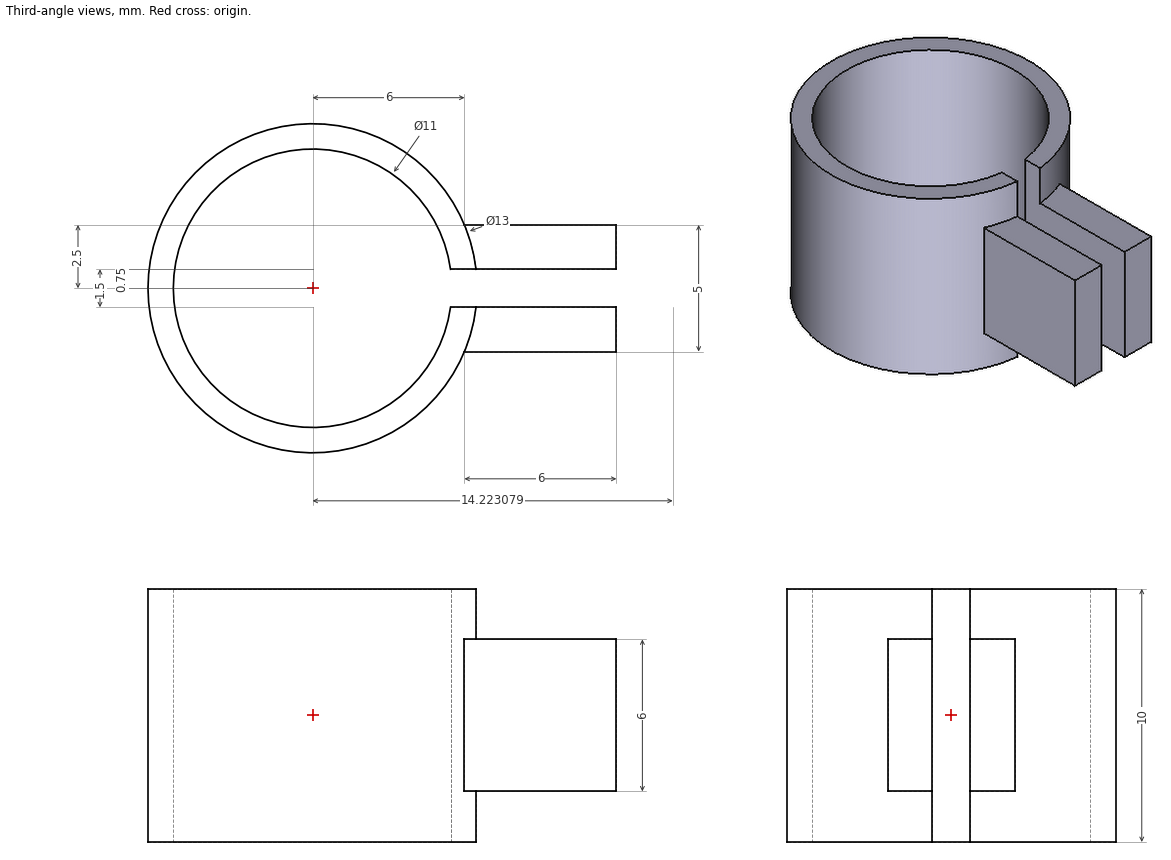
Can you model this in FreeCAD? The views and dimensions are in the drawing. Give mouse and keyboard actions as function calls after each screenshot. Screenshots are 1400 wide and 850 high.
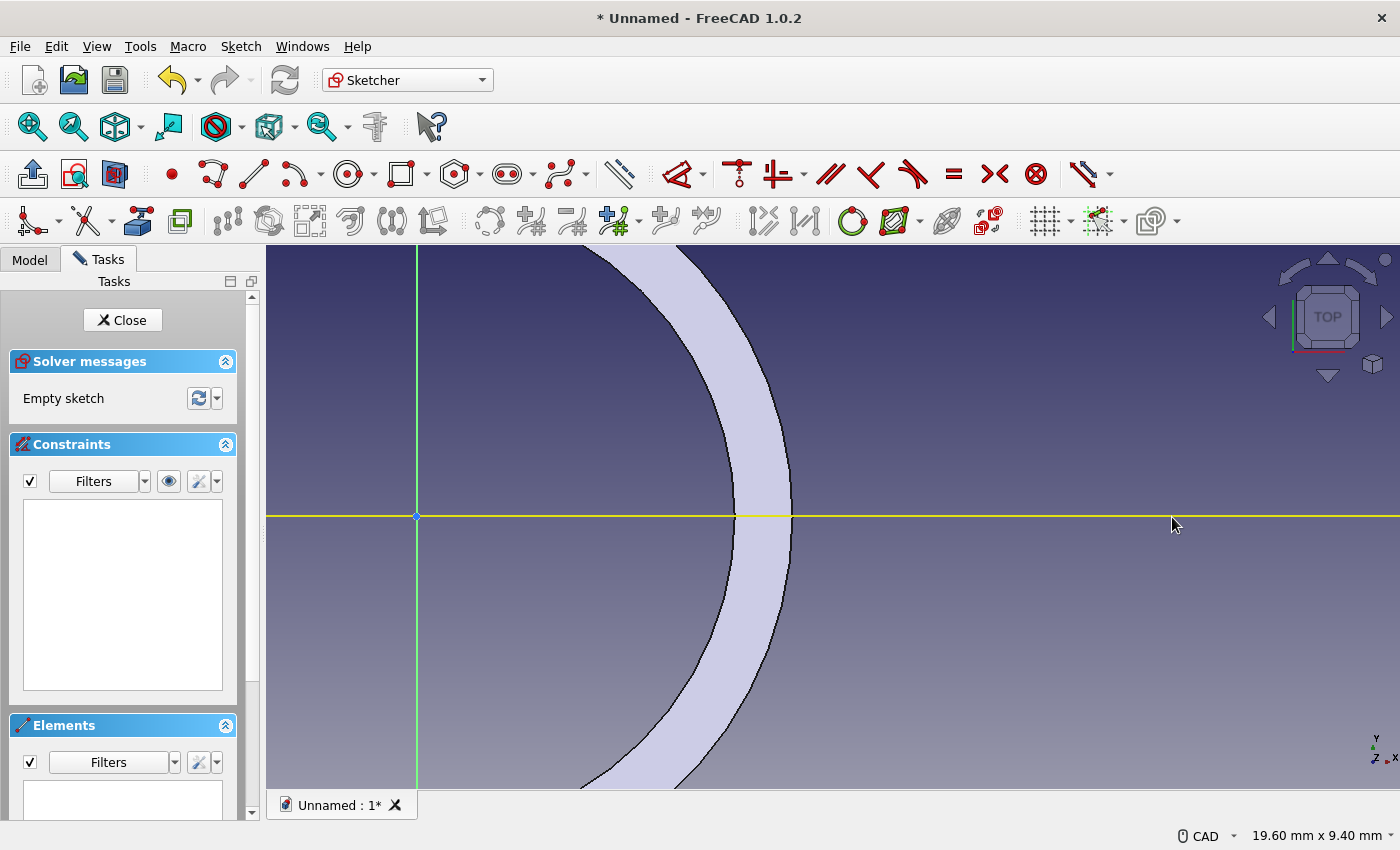
key(g)
key(r)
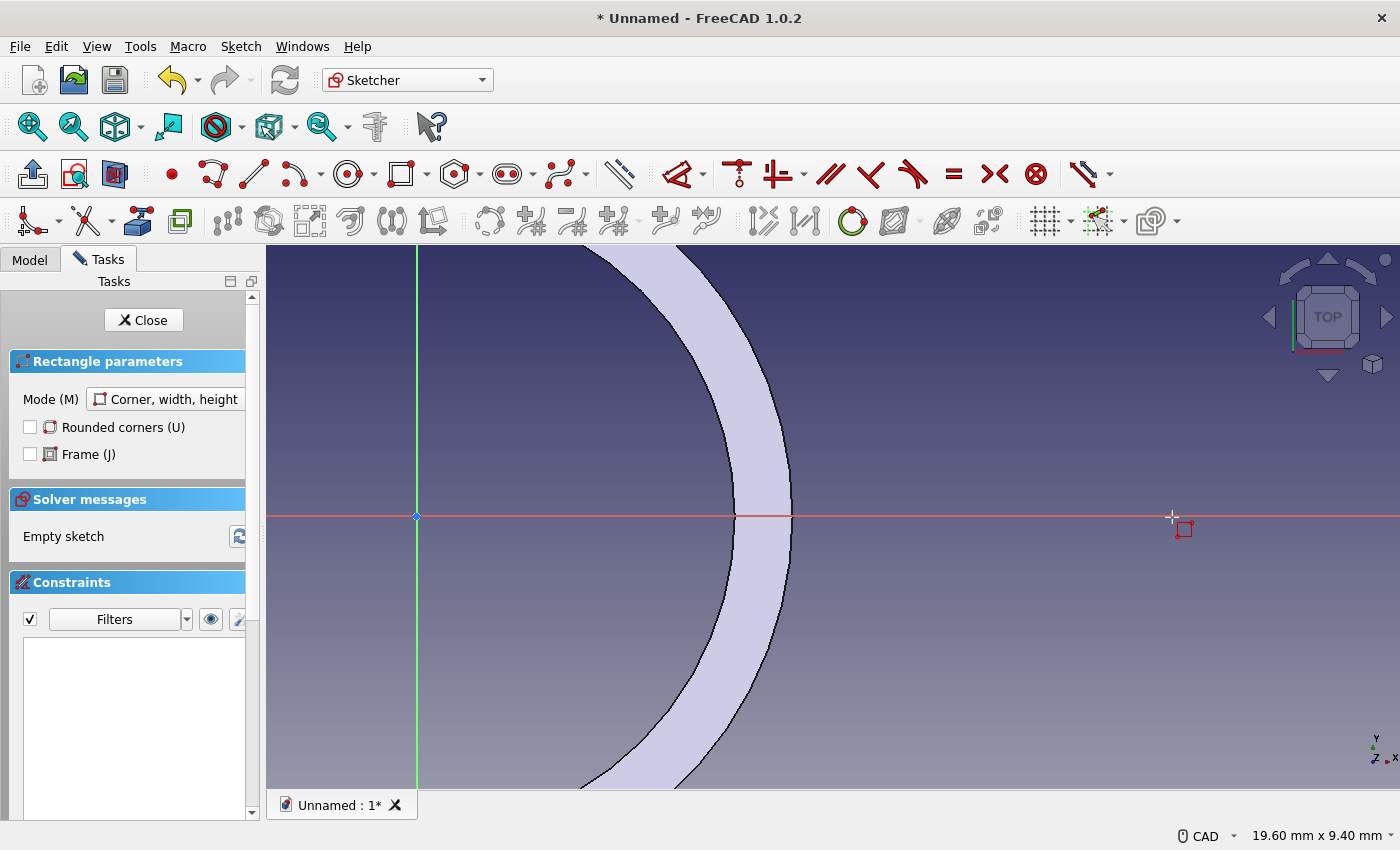
click(764, 372)
click(1111, 661)
key(Escape)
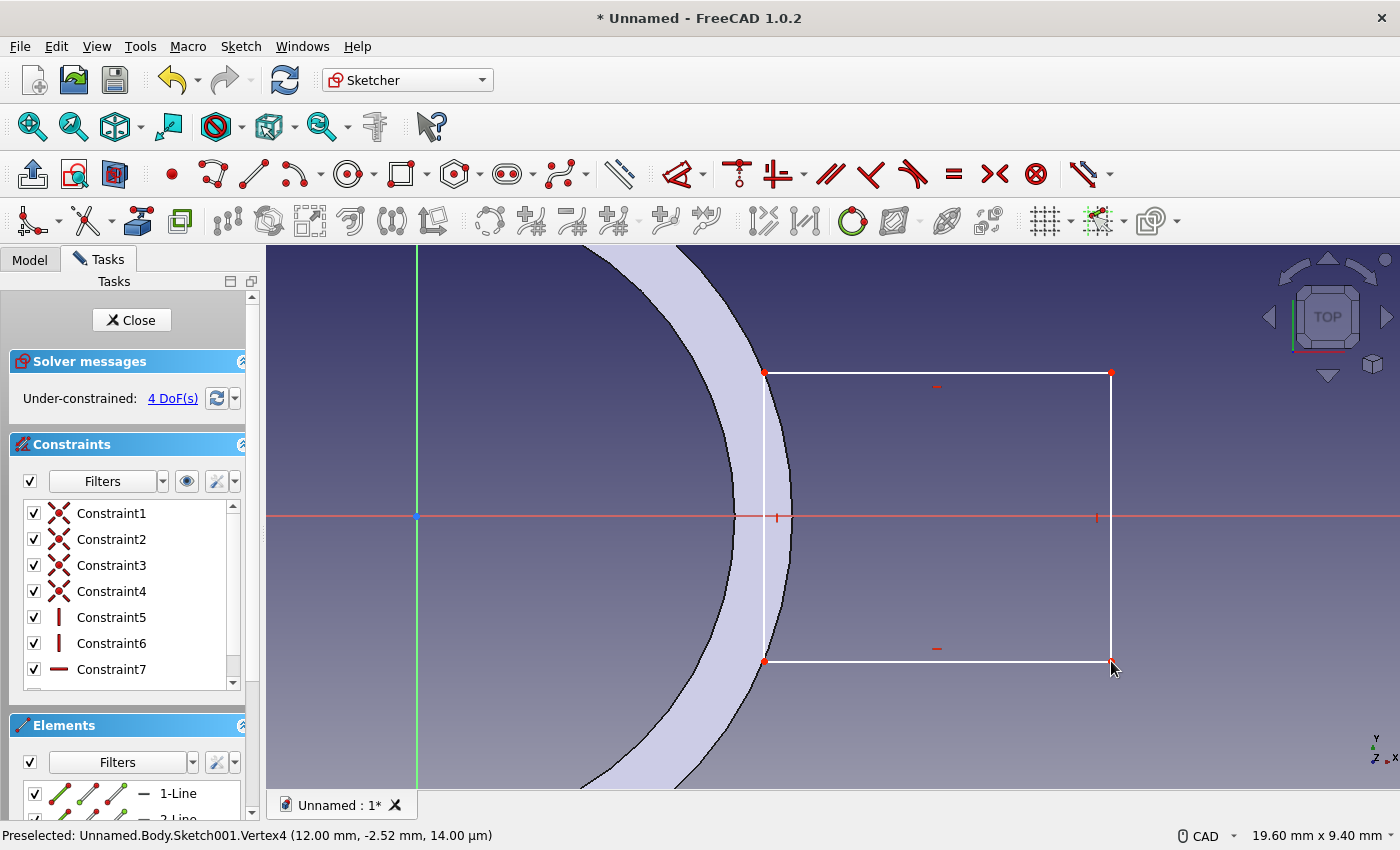
click(676, 174)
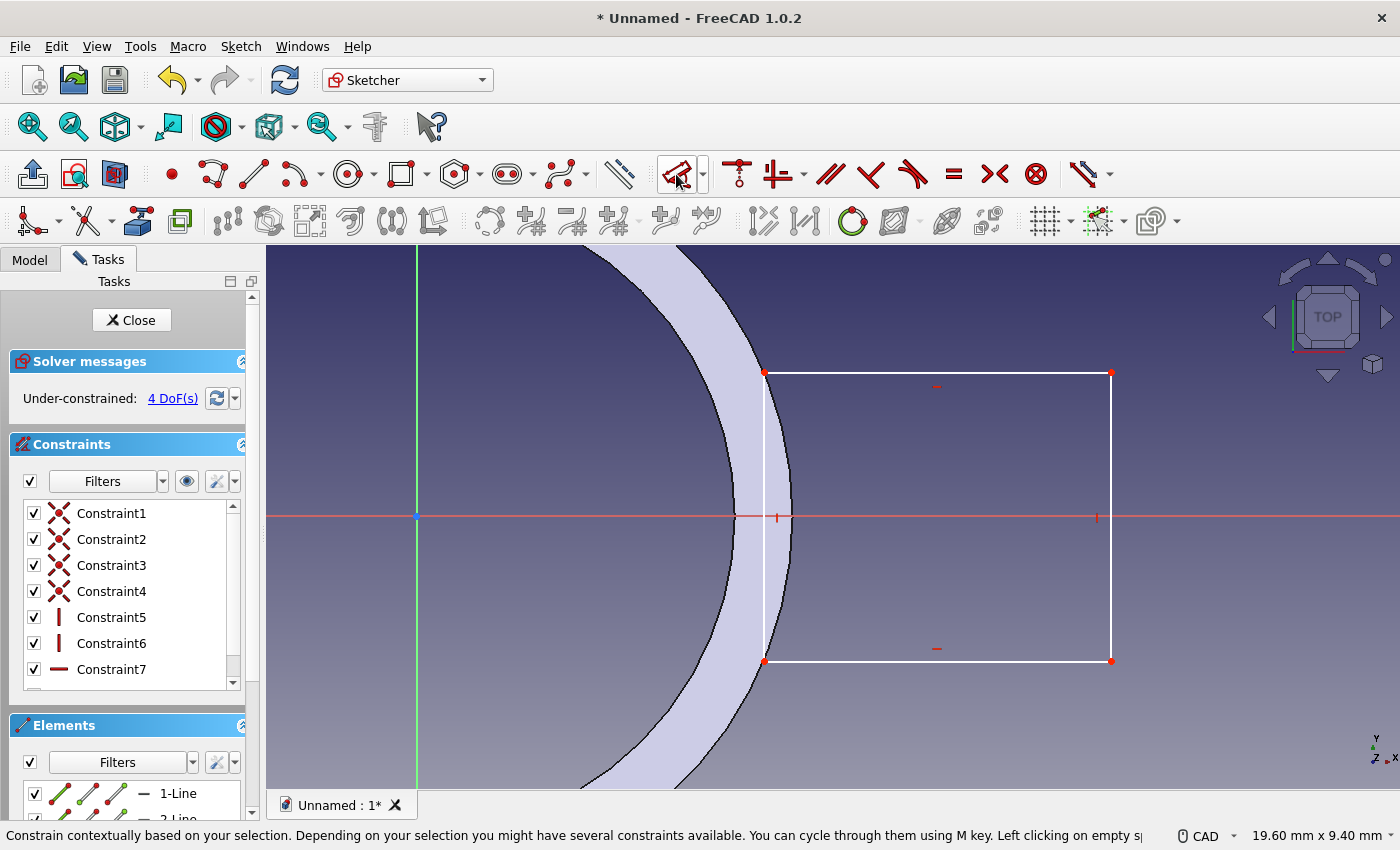
click(764, 460)
click(798, 451)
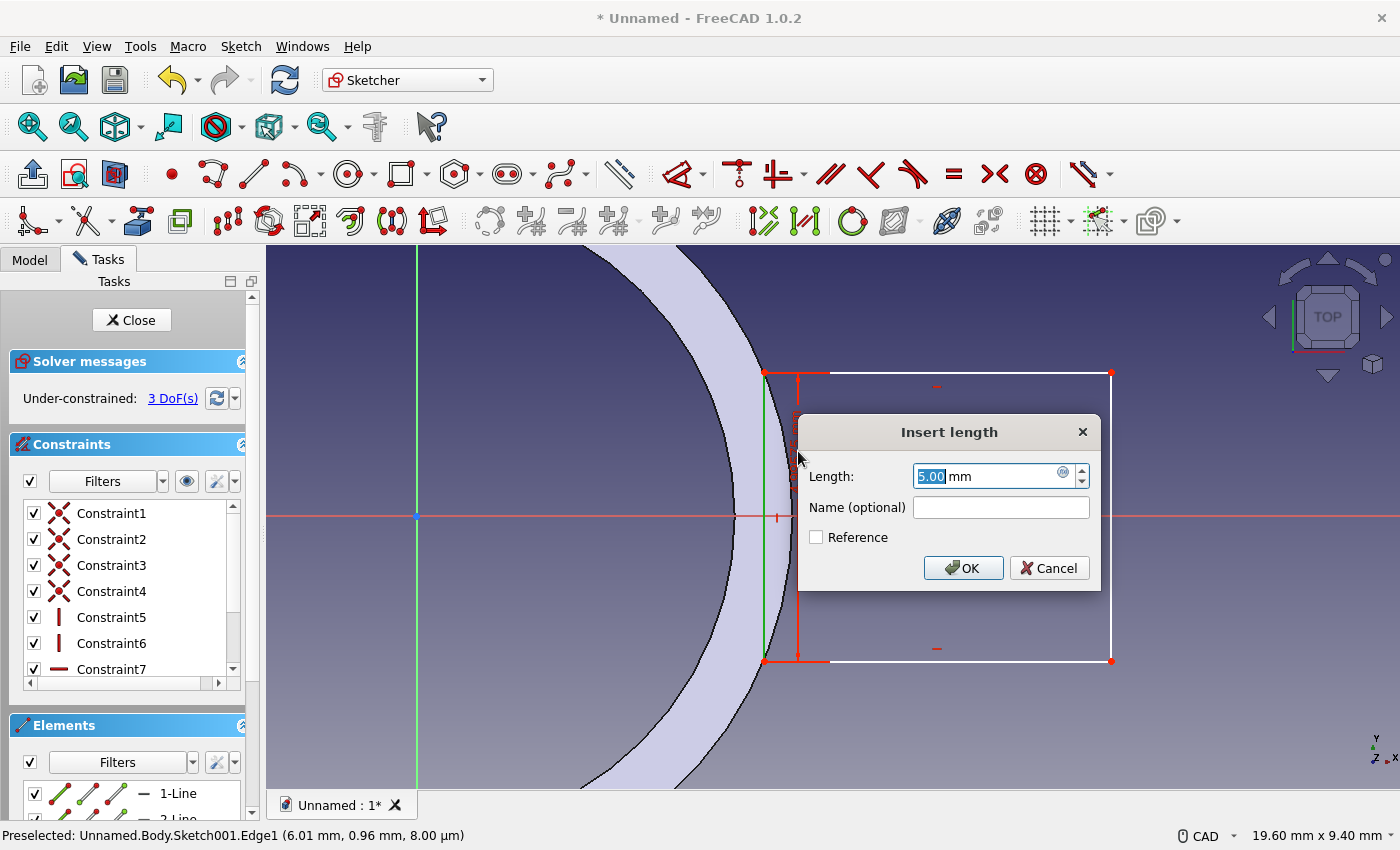
text(5)
key(Return)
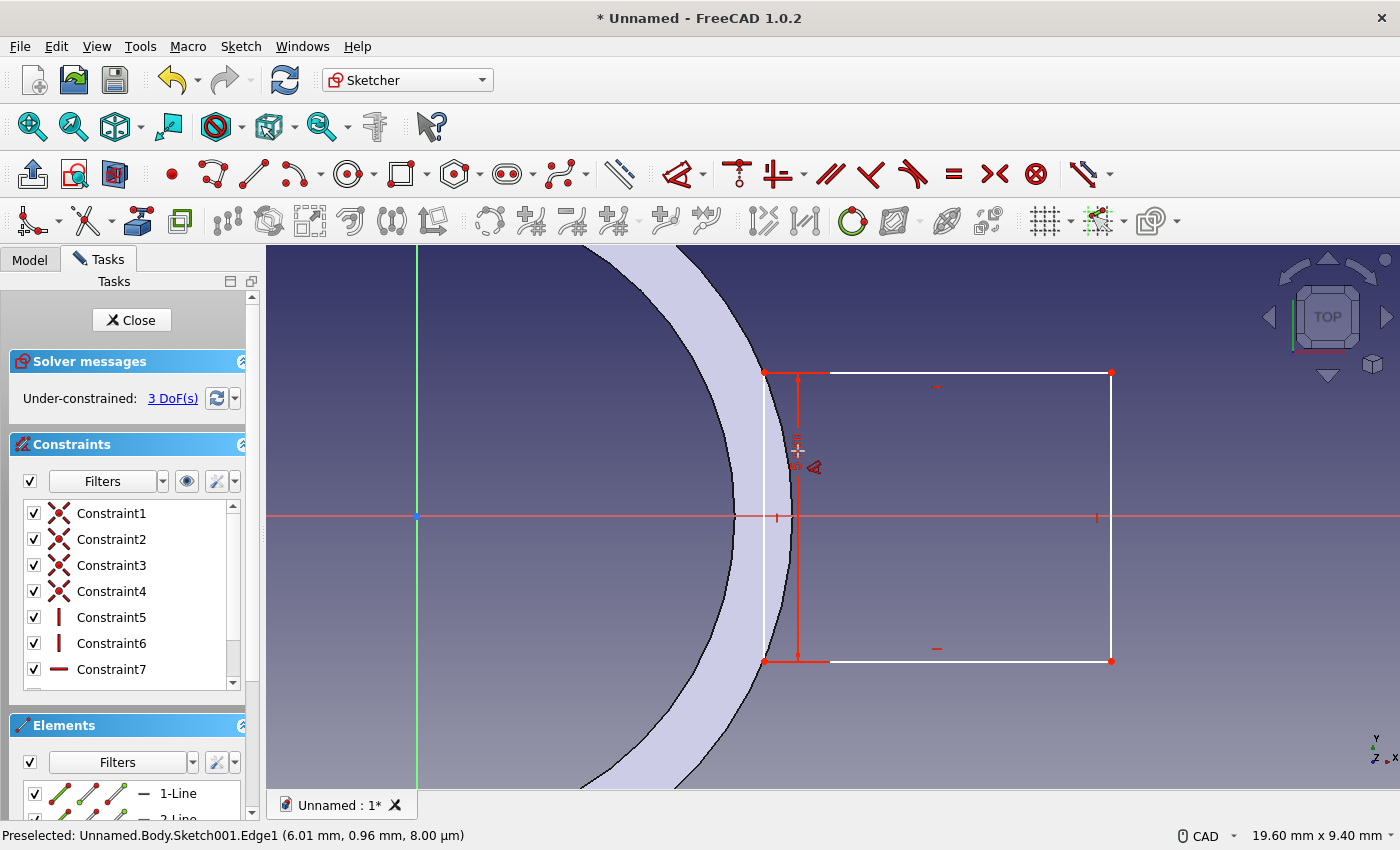
click(868, 662)
click(937, 696)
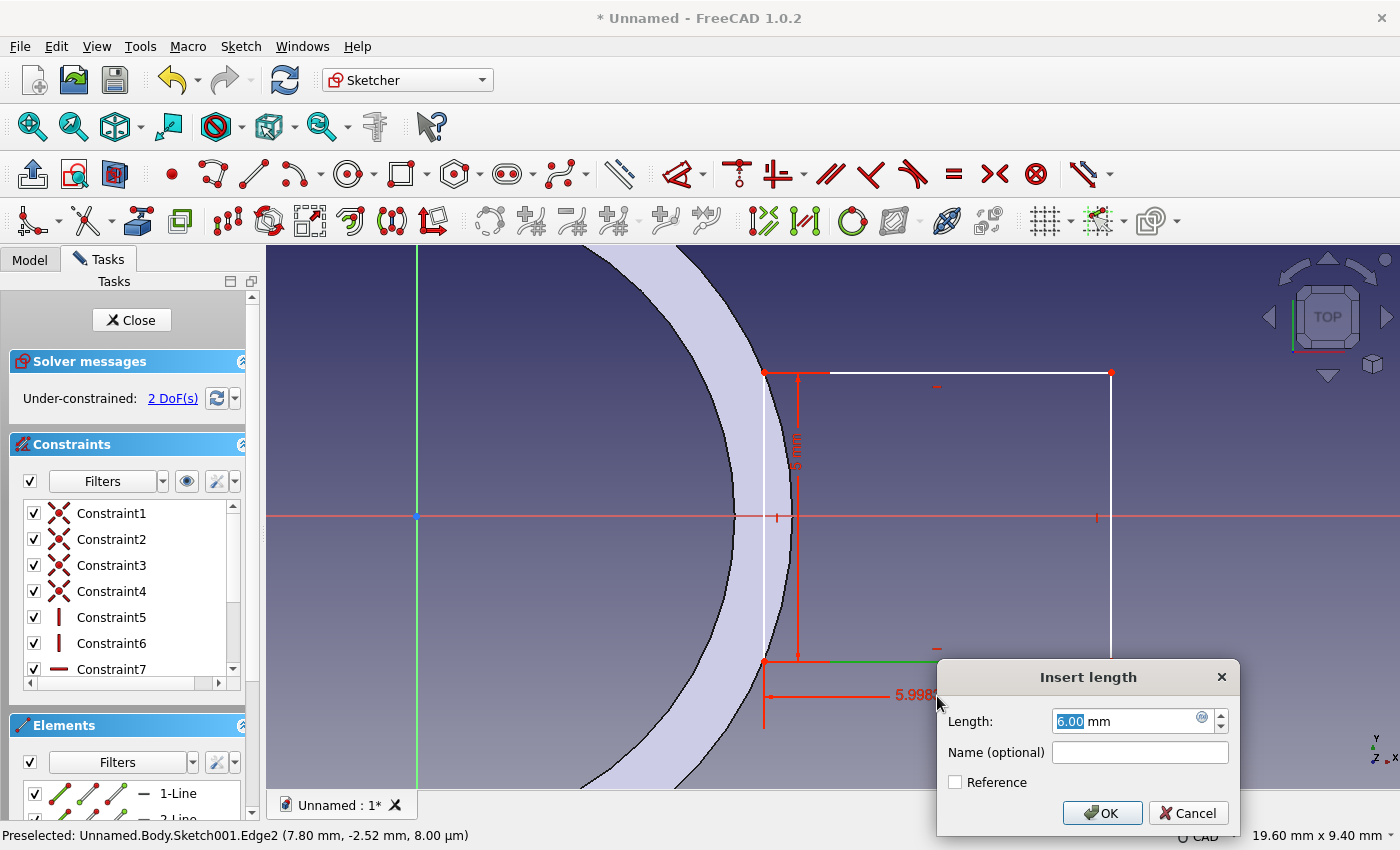
text(6)
key(Return)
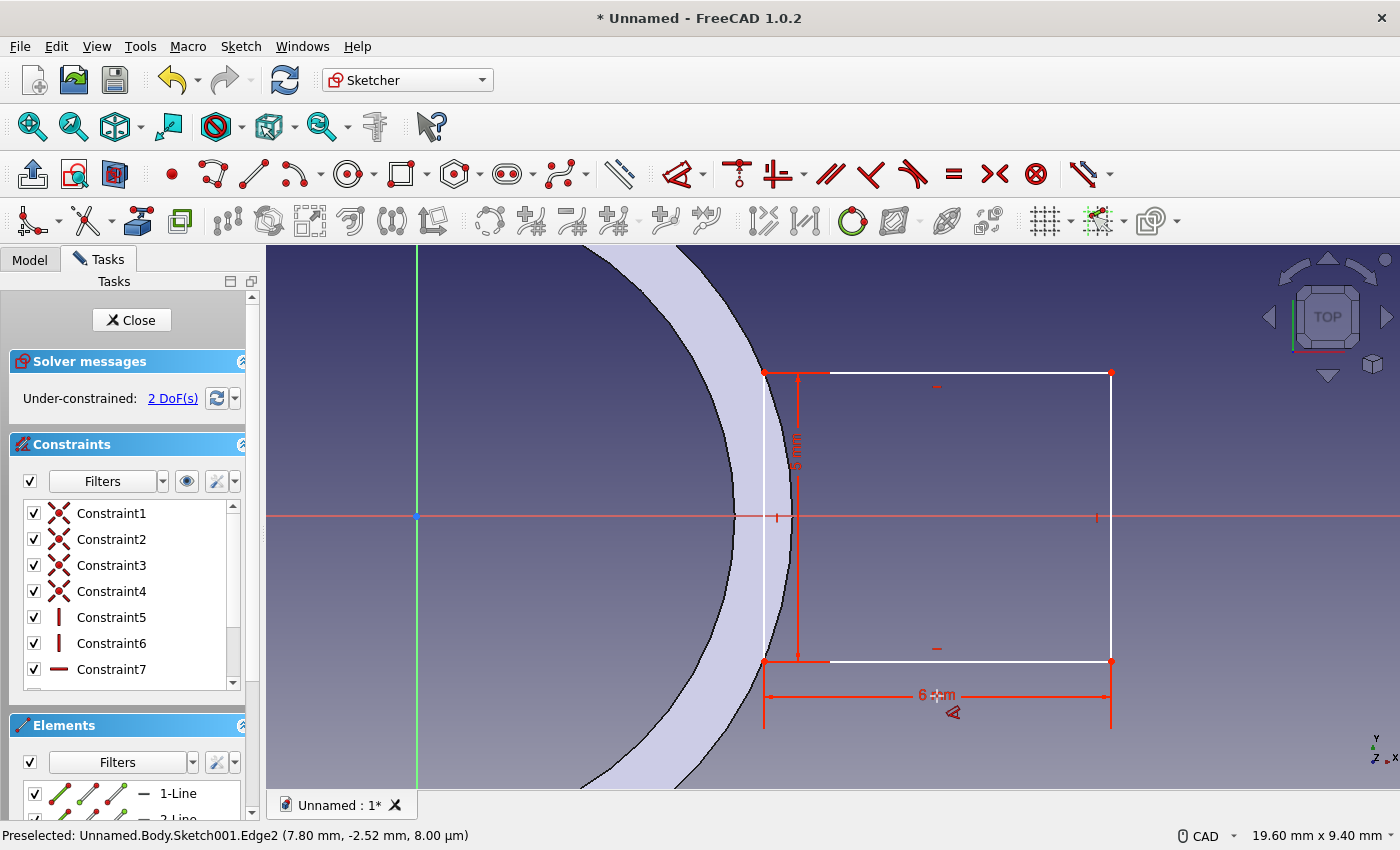
click(764, 373)
click(590, 339)